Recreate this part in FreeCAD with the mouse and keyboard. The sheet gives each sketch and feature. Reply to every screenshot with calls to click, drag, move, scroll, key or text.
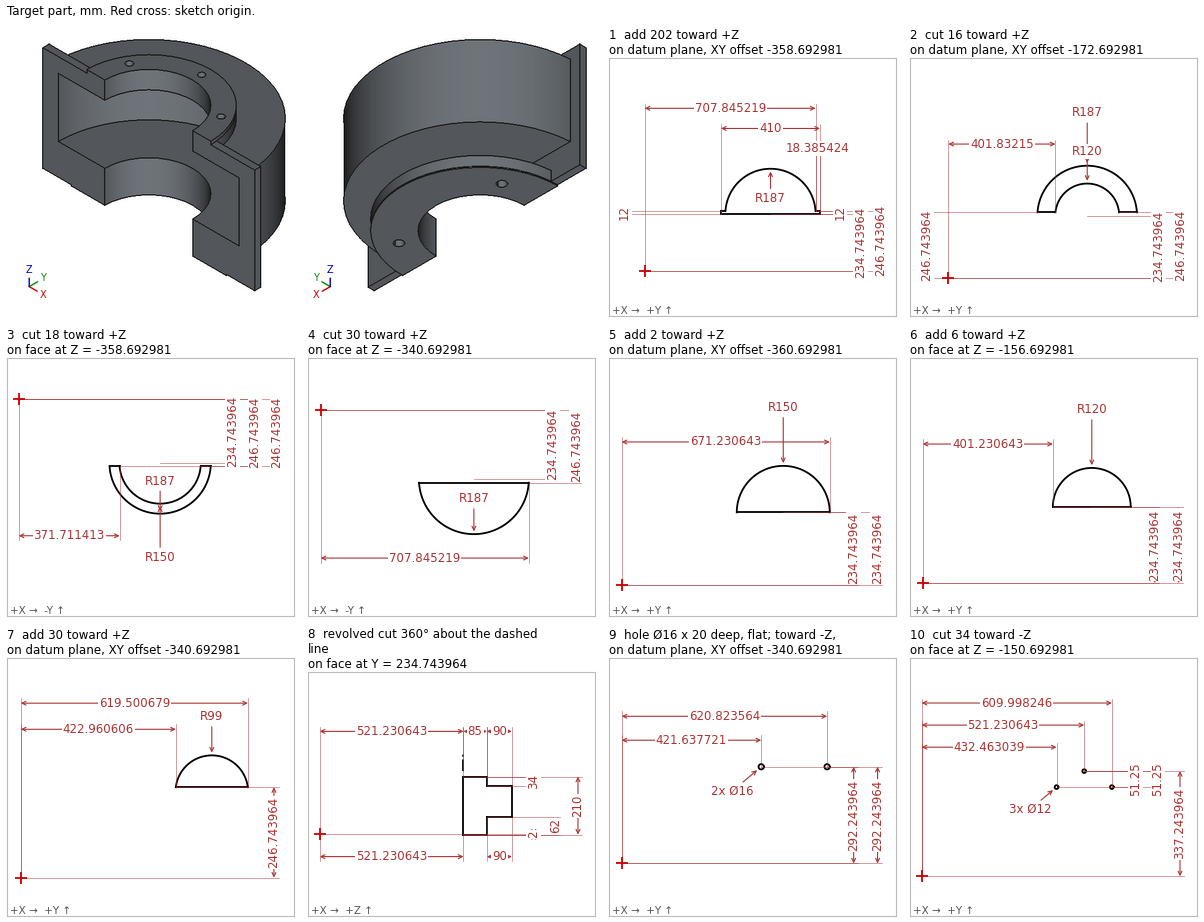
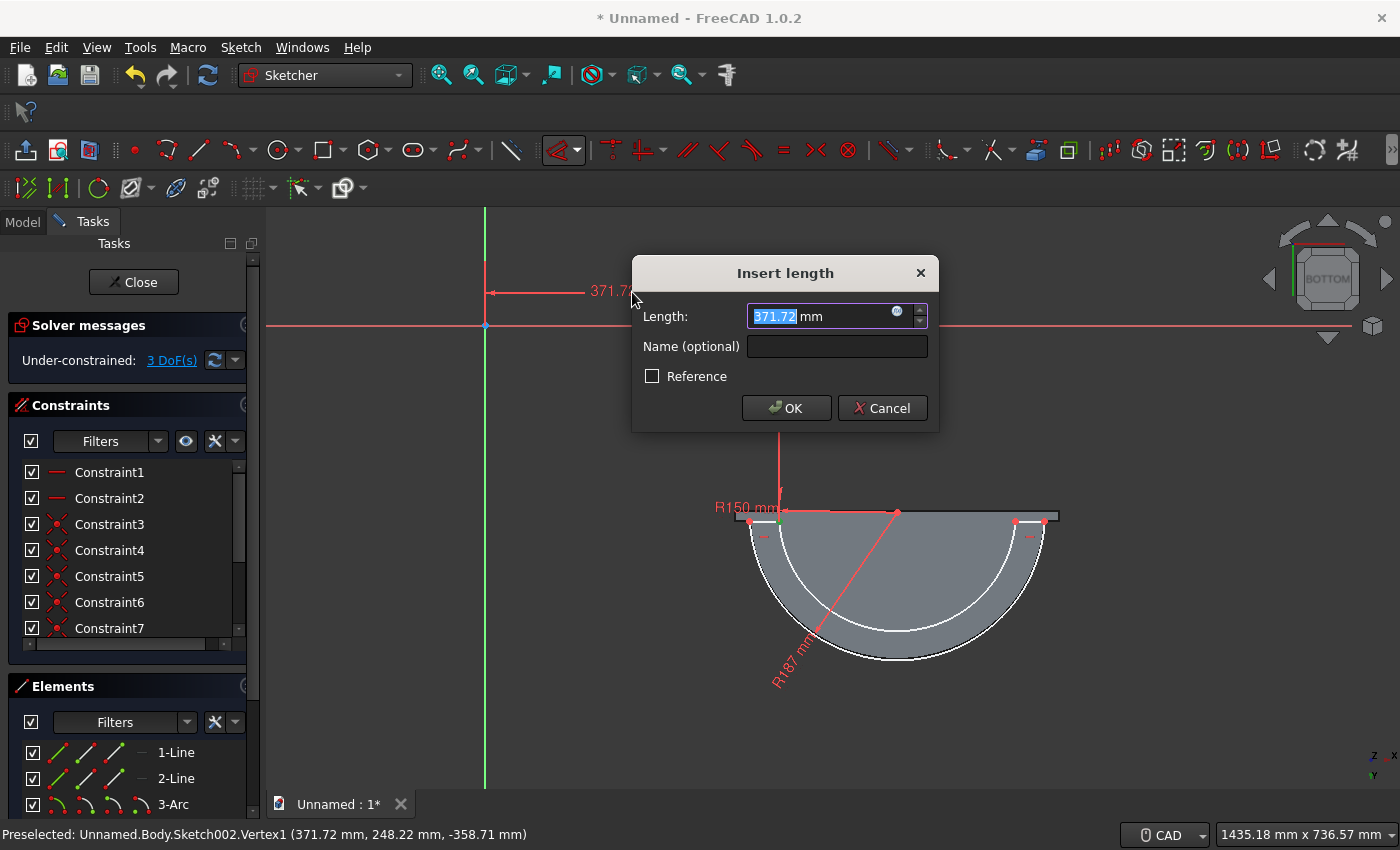
text(371.711413)
key(Return)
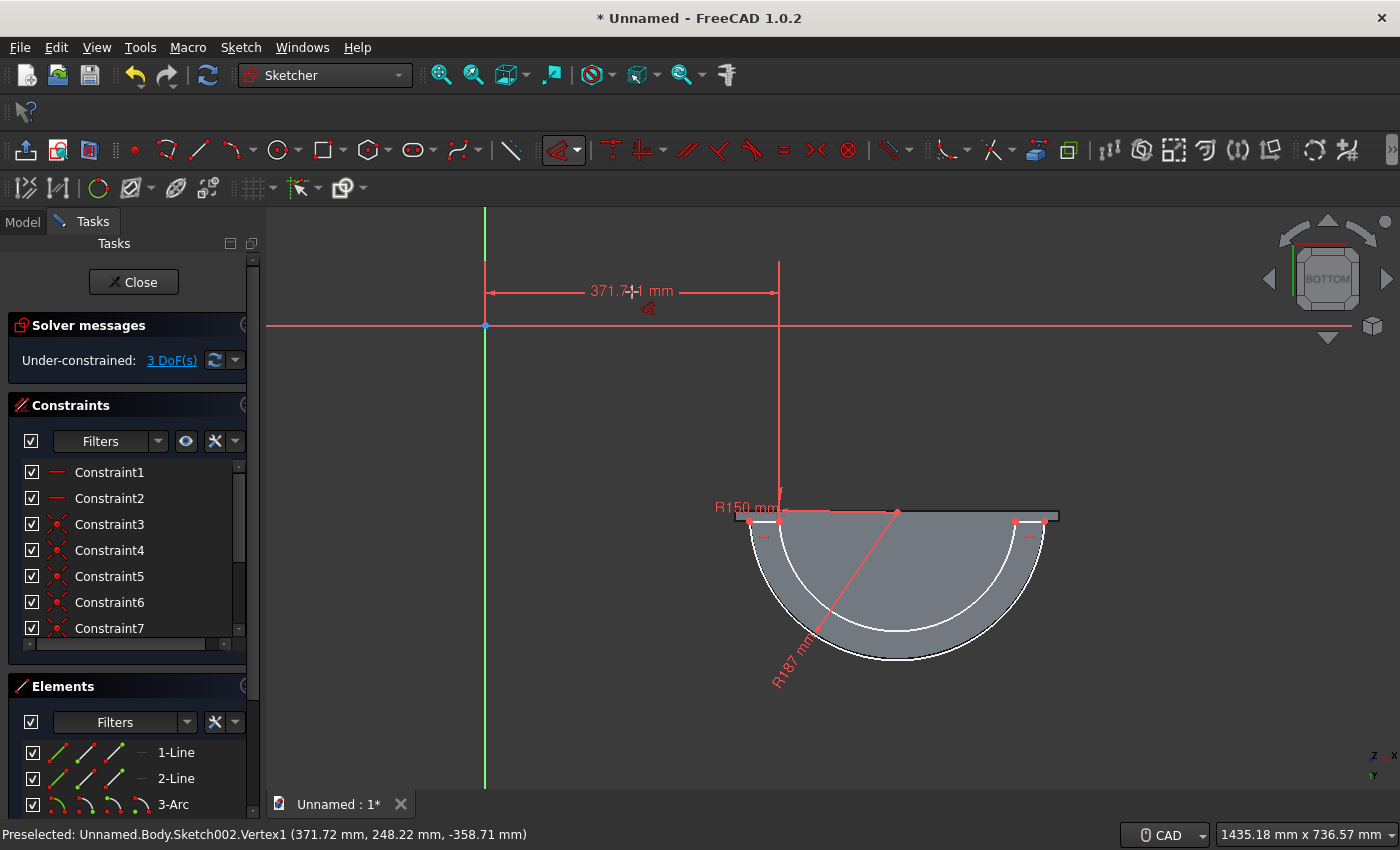
click(779, 522)
click(451, 424)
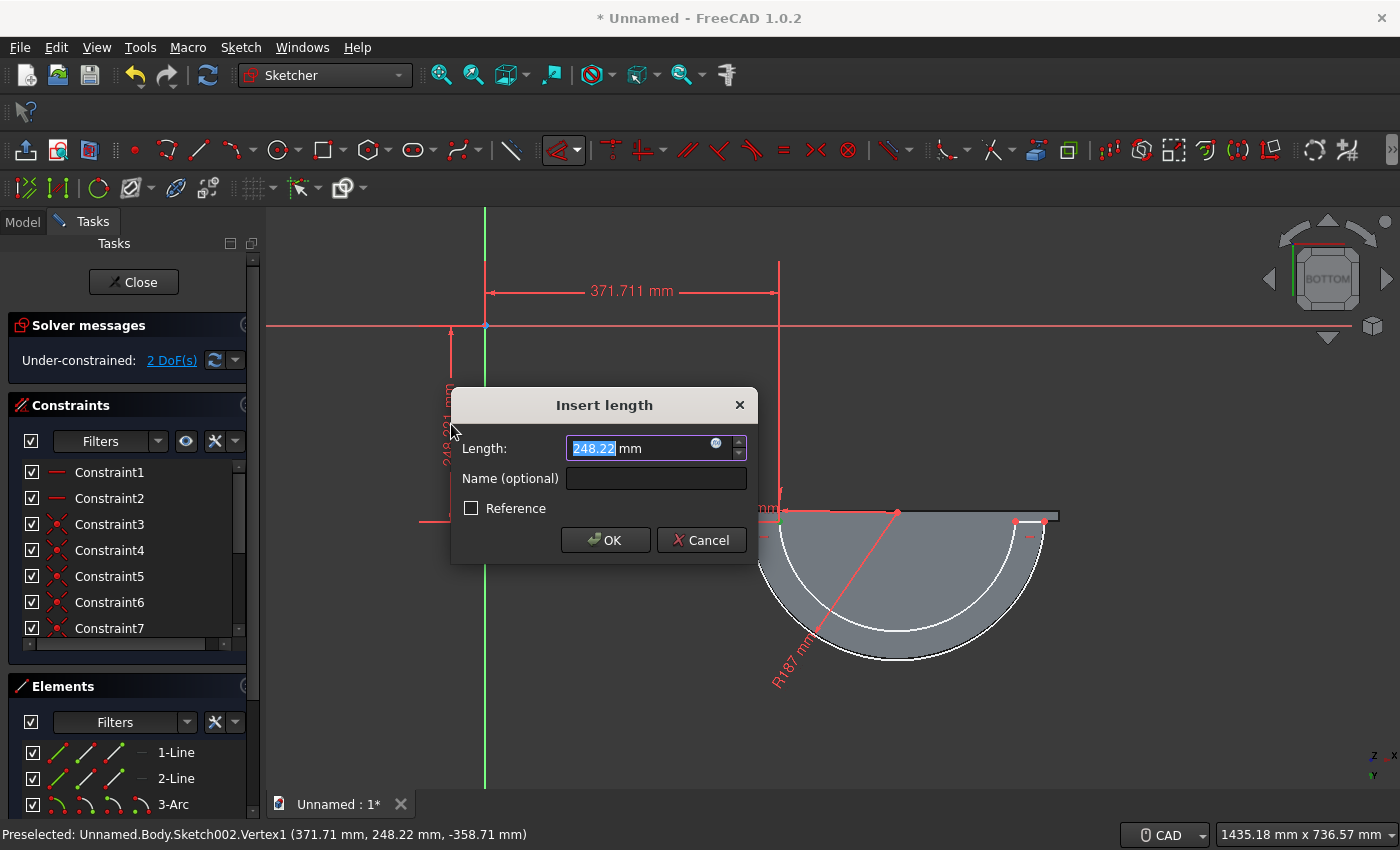
text(246.743964)
key(Return)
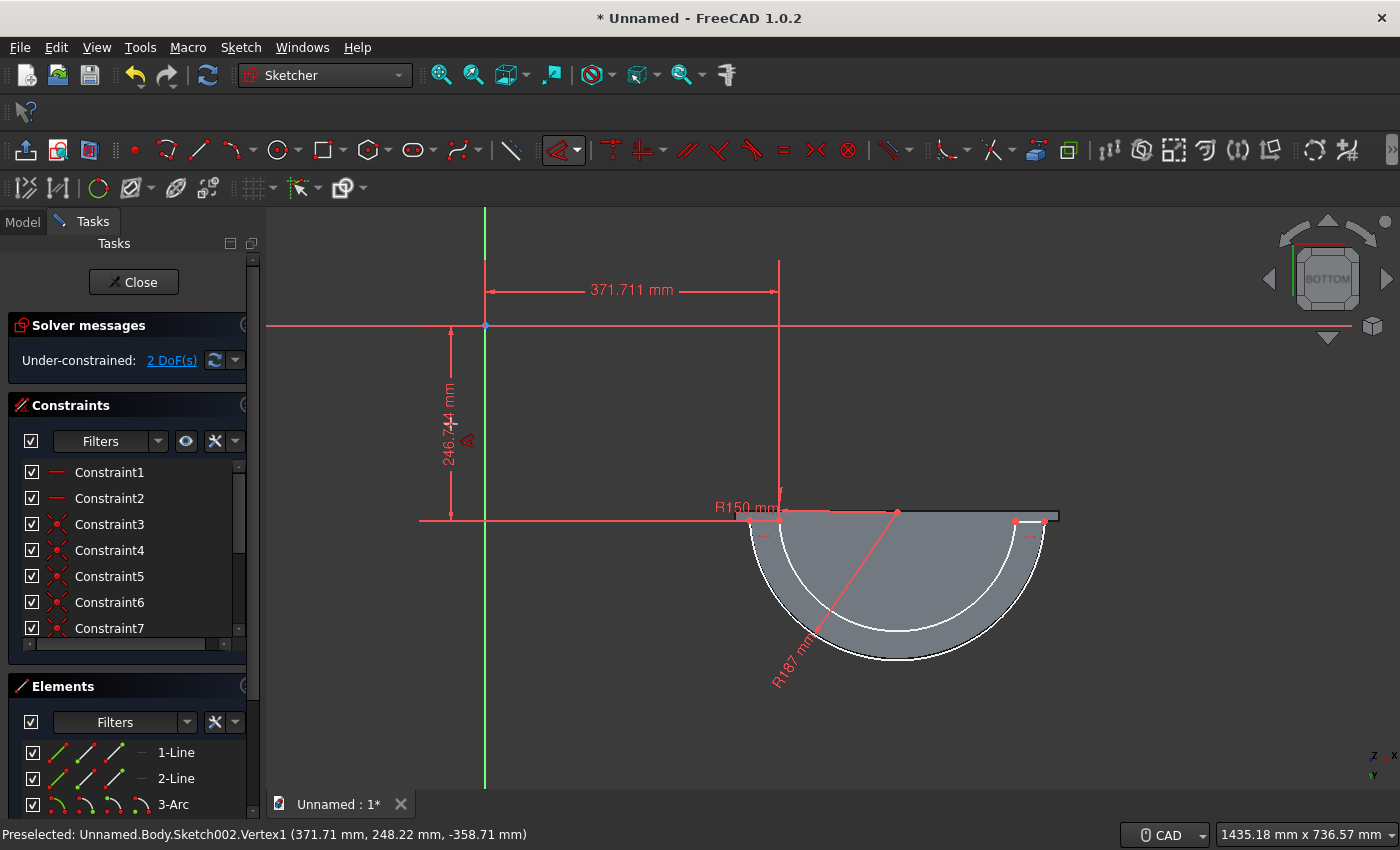
click(1045, 522)
click(1079, 424)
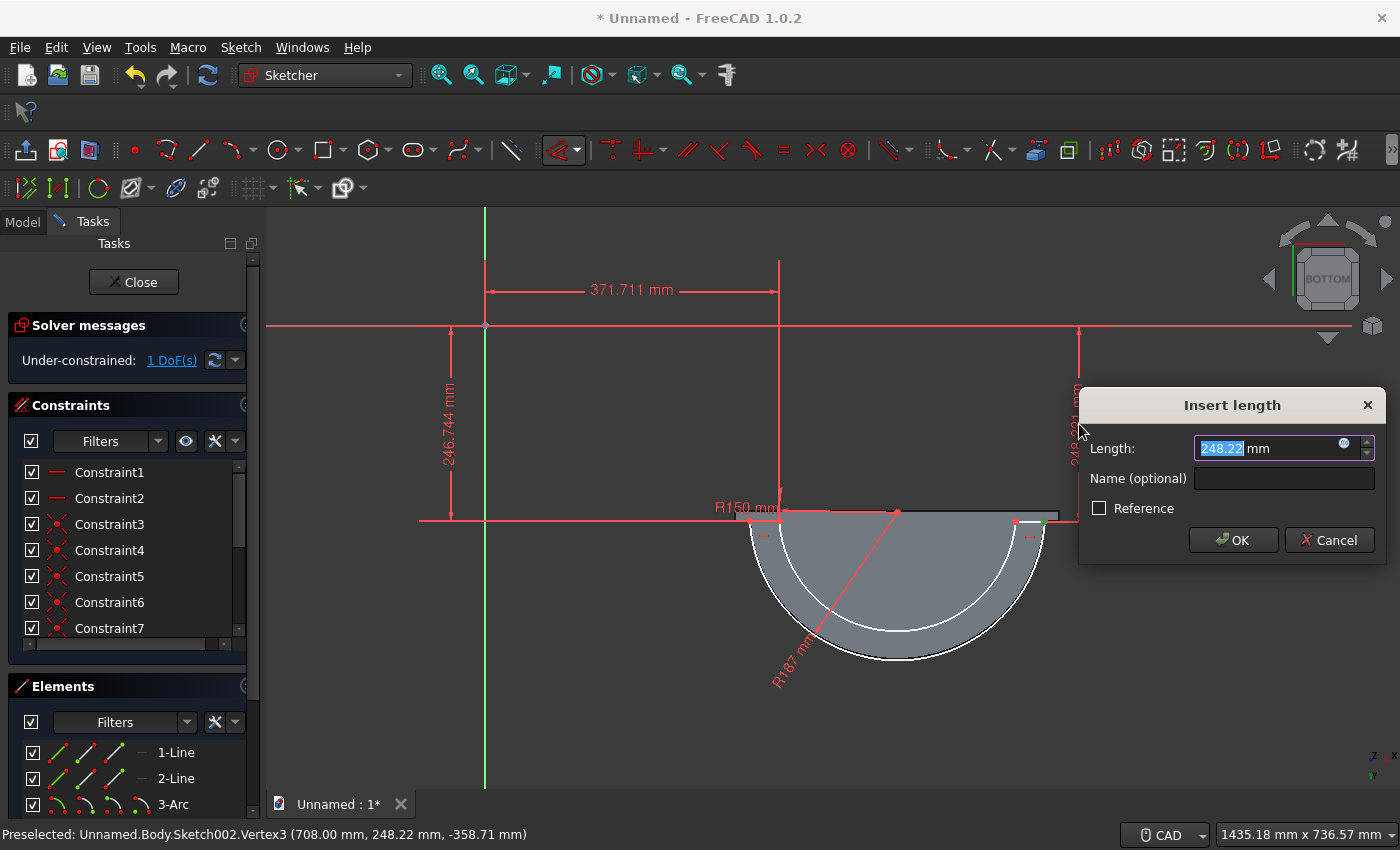
text(246.743964)
key(Return)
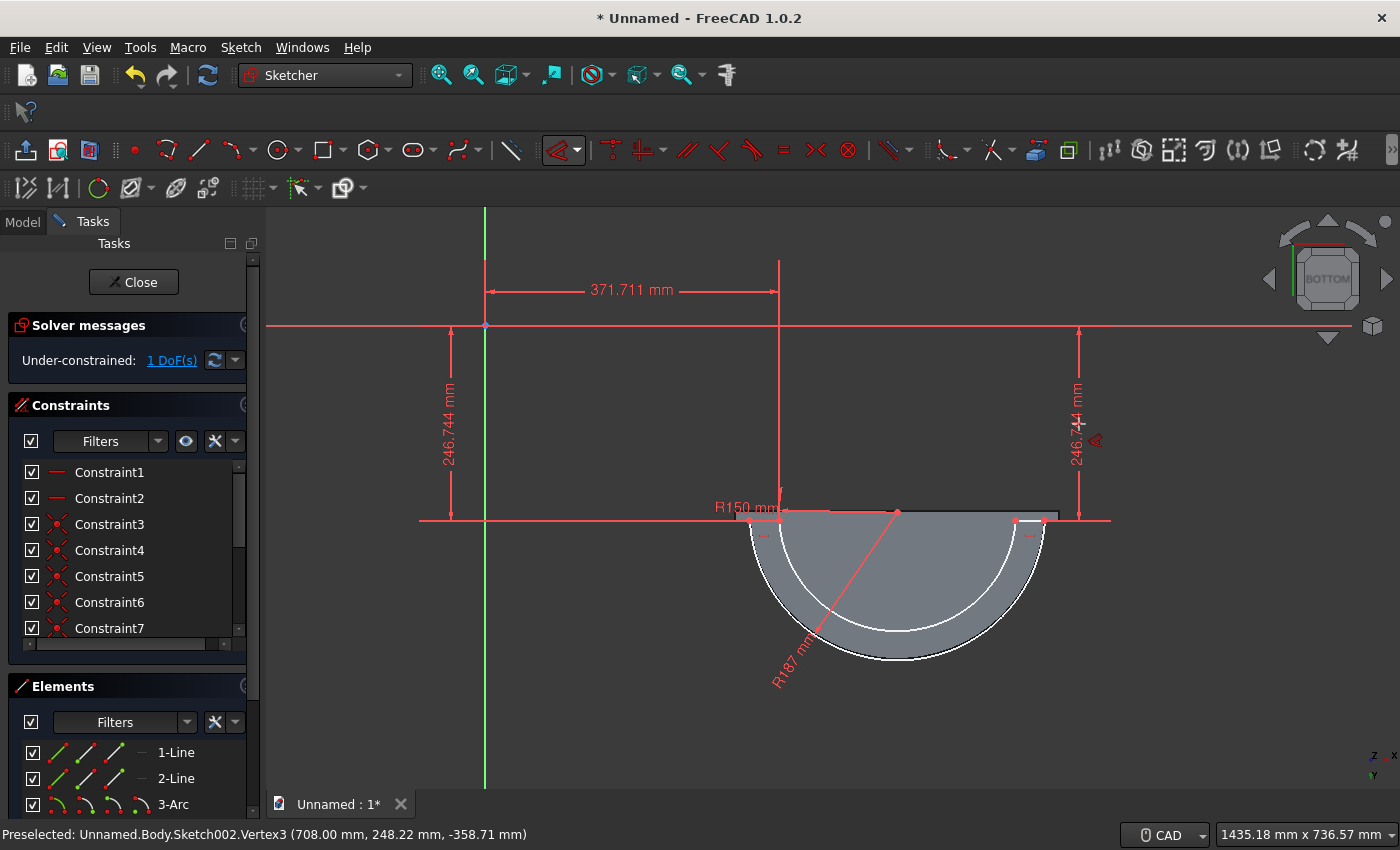
click(897, 513)
click(451, 376)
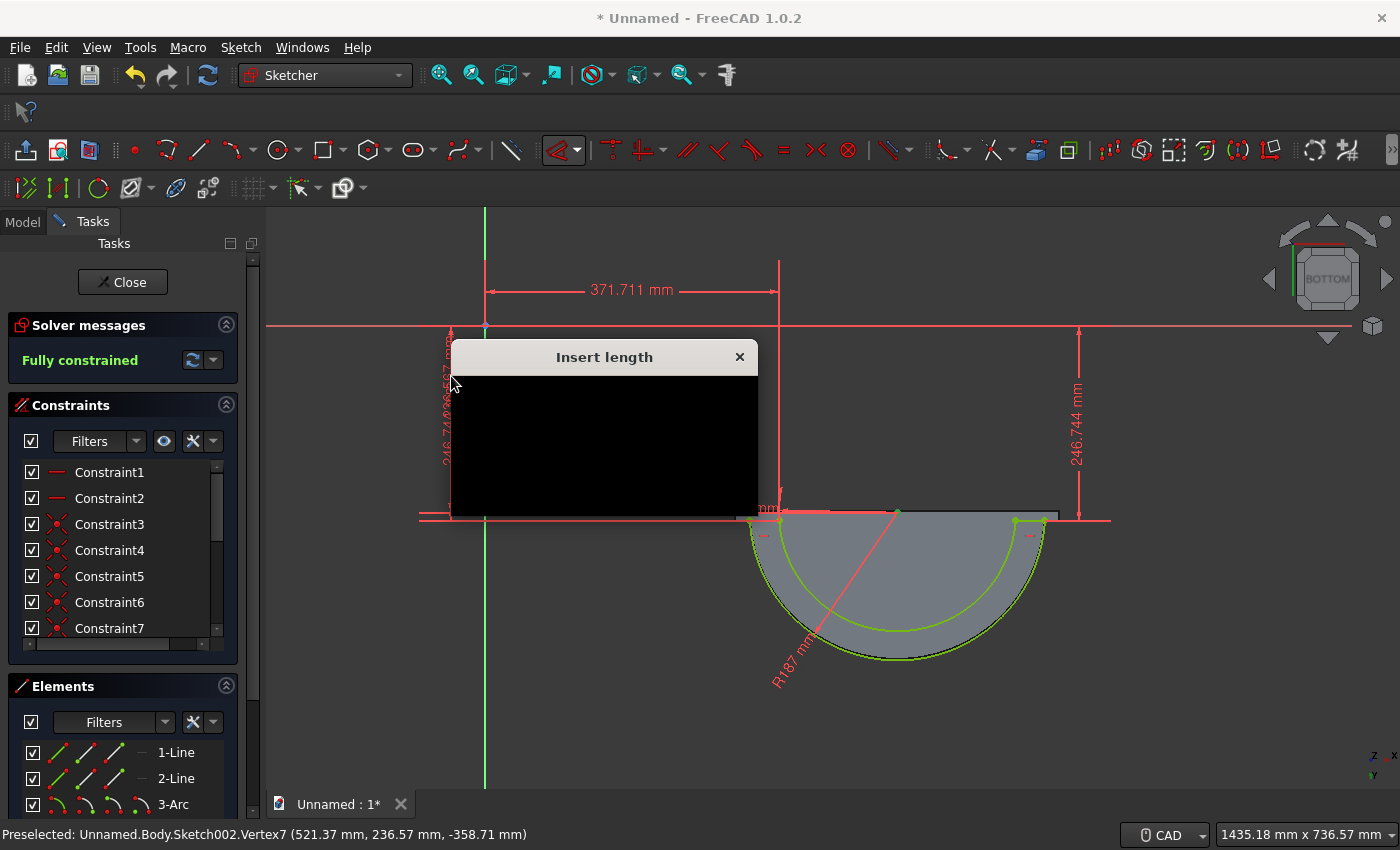
text(234.743964)
key(Return)
key(Escape)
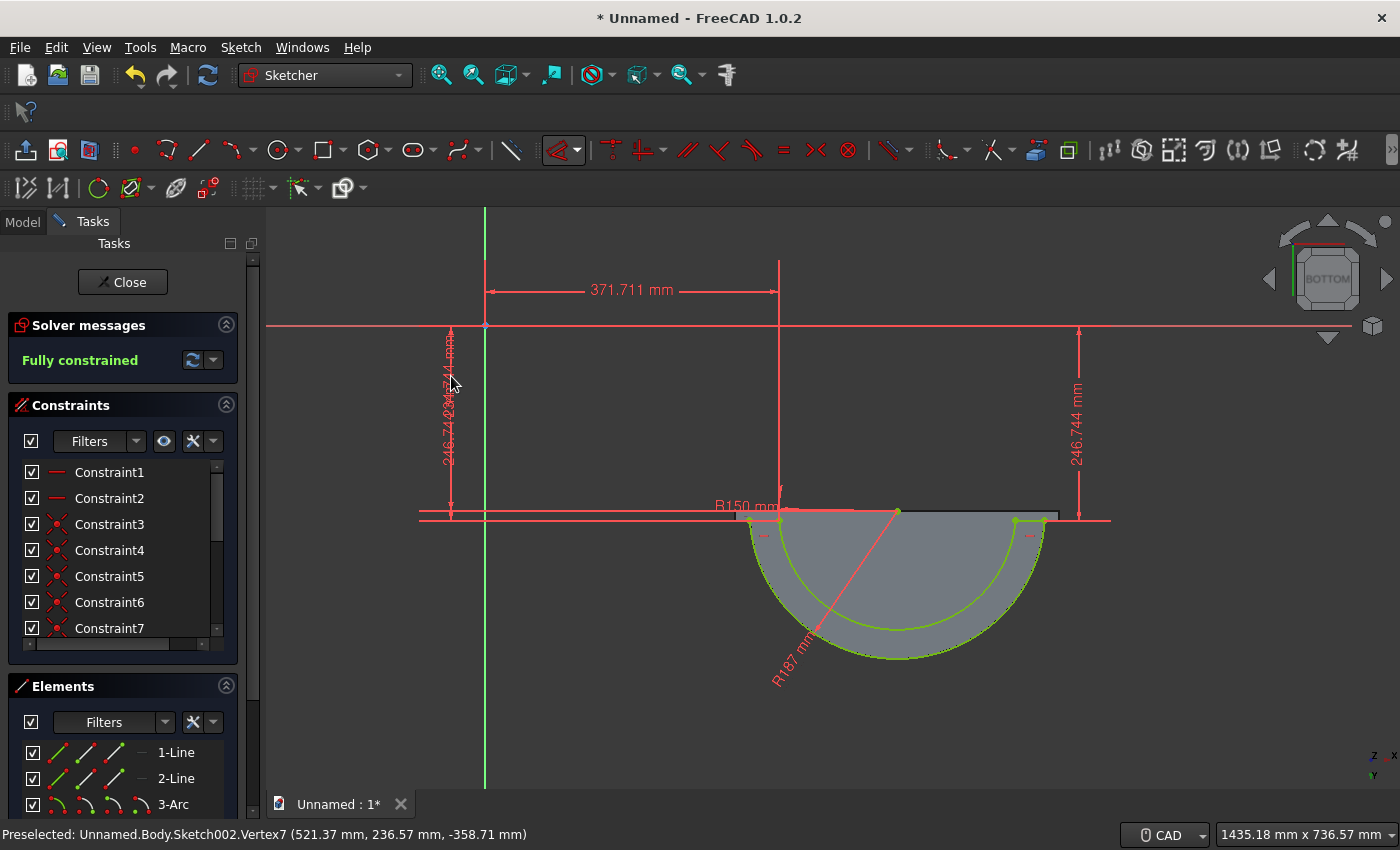
click(123, 282)